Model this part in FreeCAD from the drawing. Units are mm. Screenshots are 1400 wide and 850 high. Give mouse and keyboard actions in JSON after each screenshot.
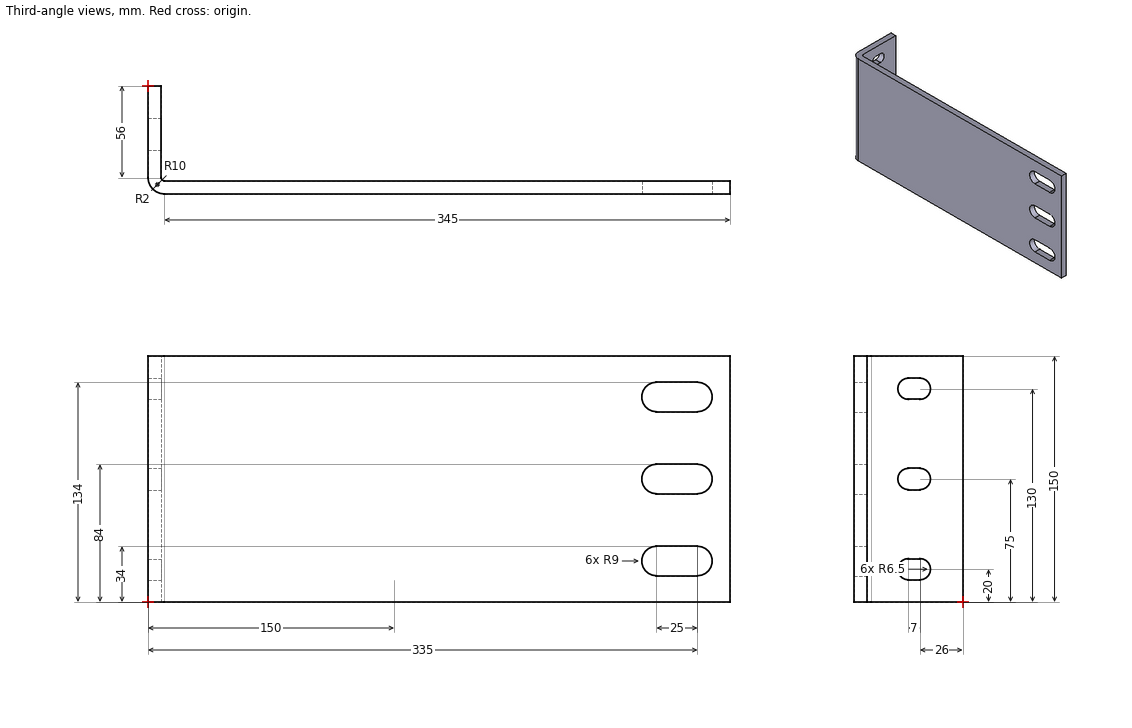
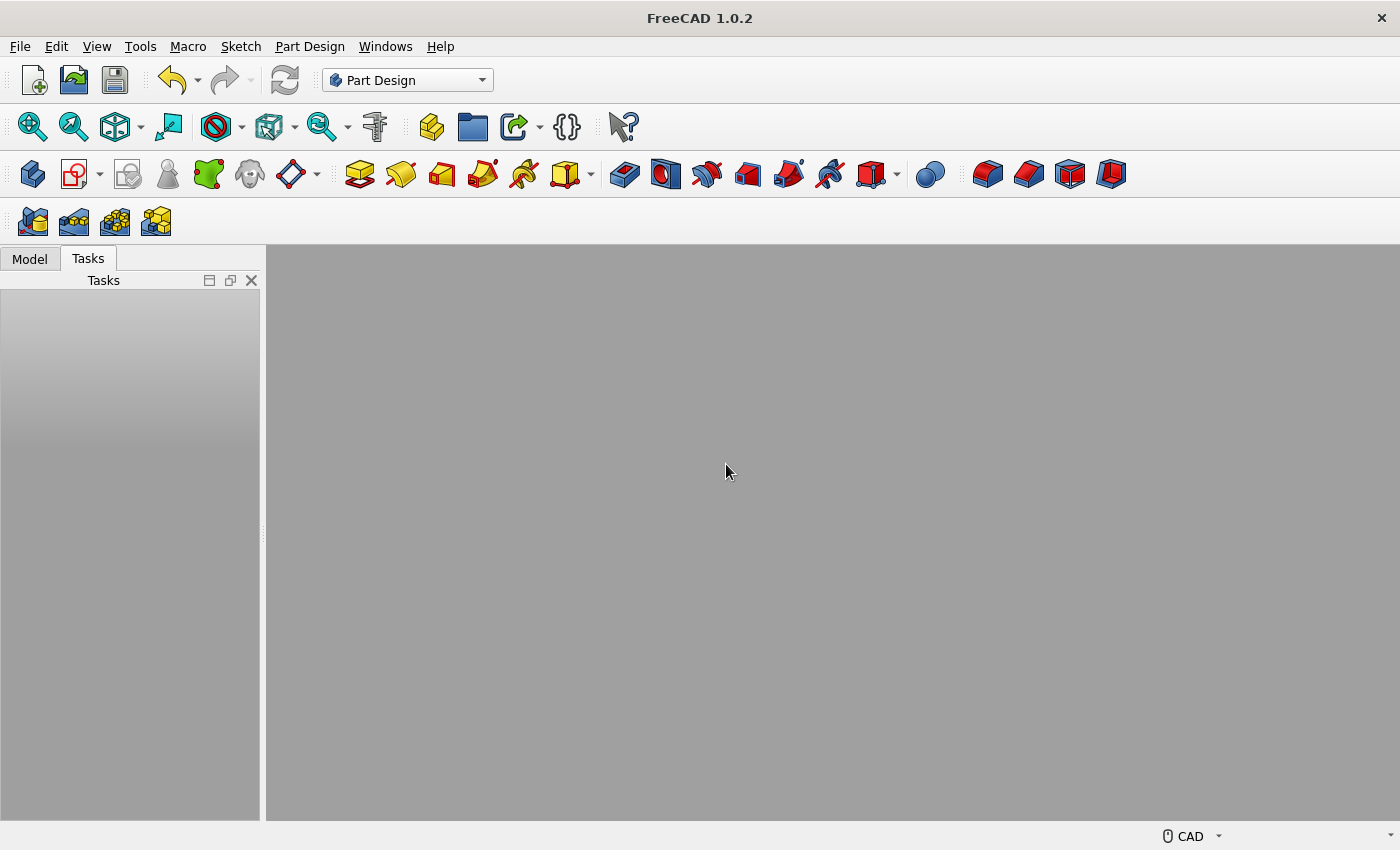
{"action": "left_click", "coordinate": [33, 80]}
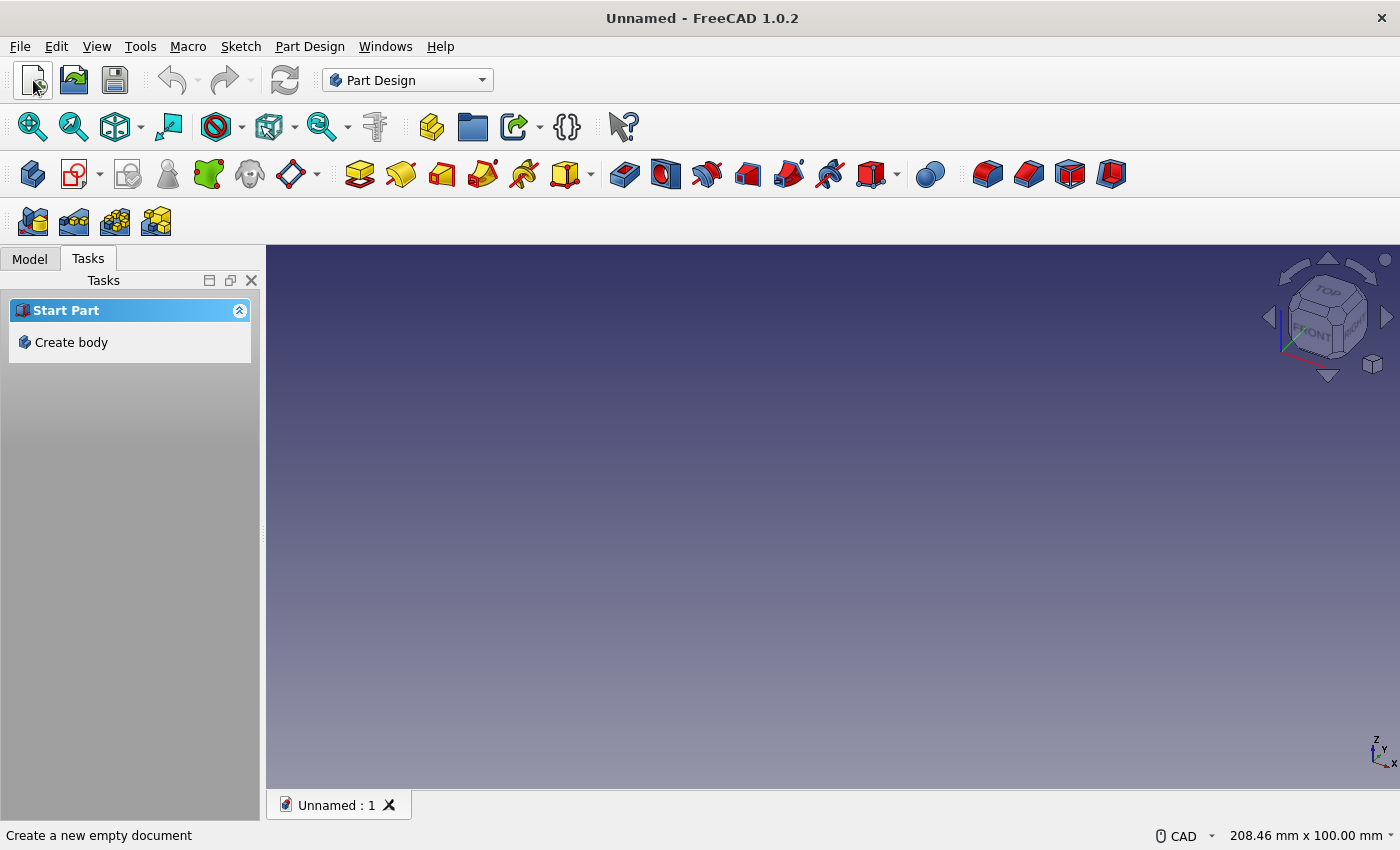
{"action": "left_click", "coordinate": [74, 174]}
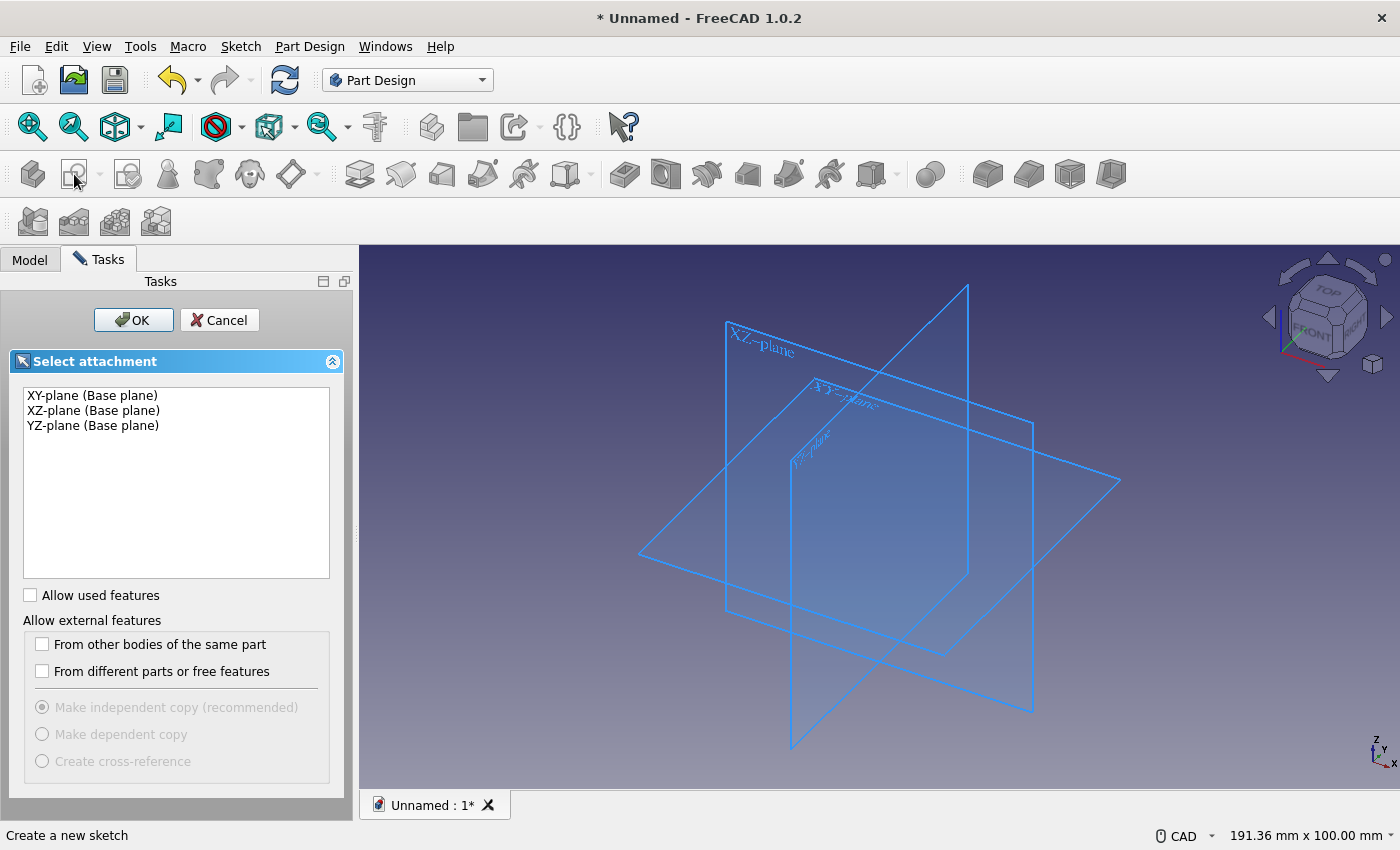
{"action": "left_click", "coordinate": [84, 396]}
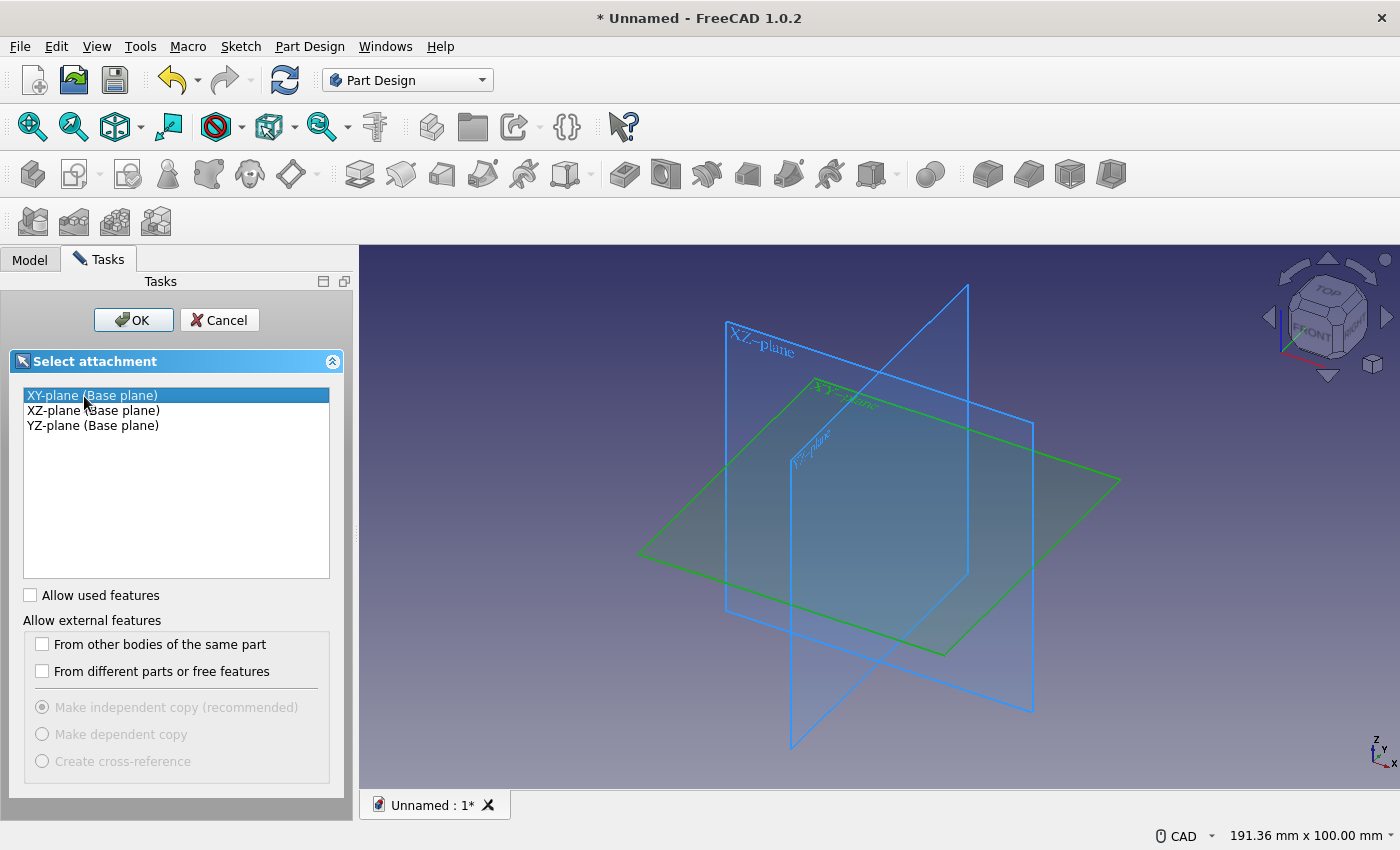
{"action": "left_click", "coordinate": [134, 320]}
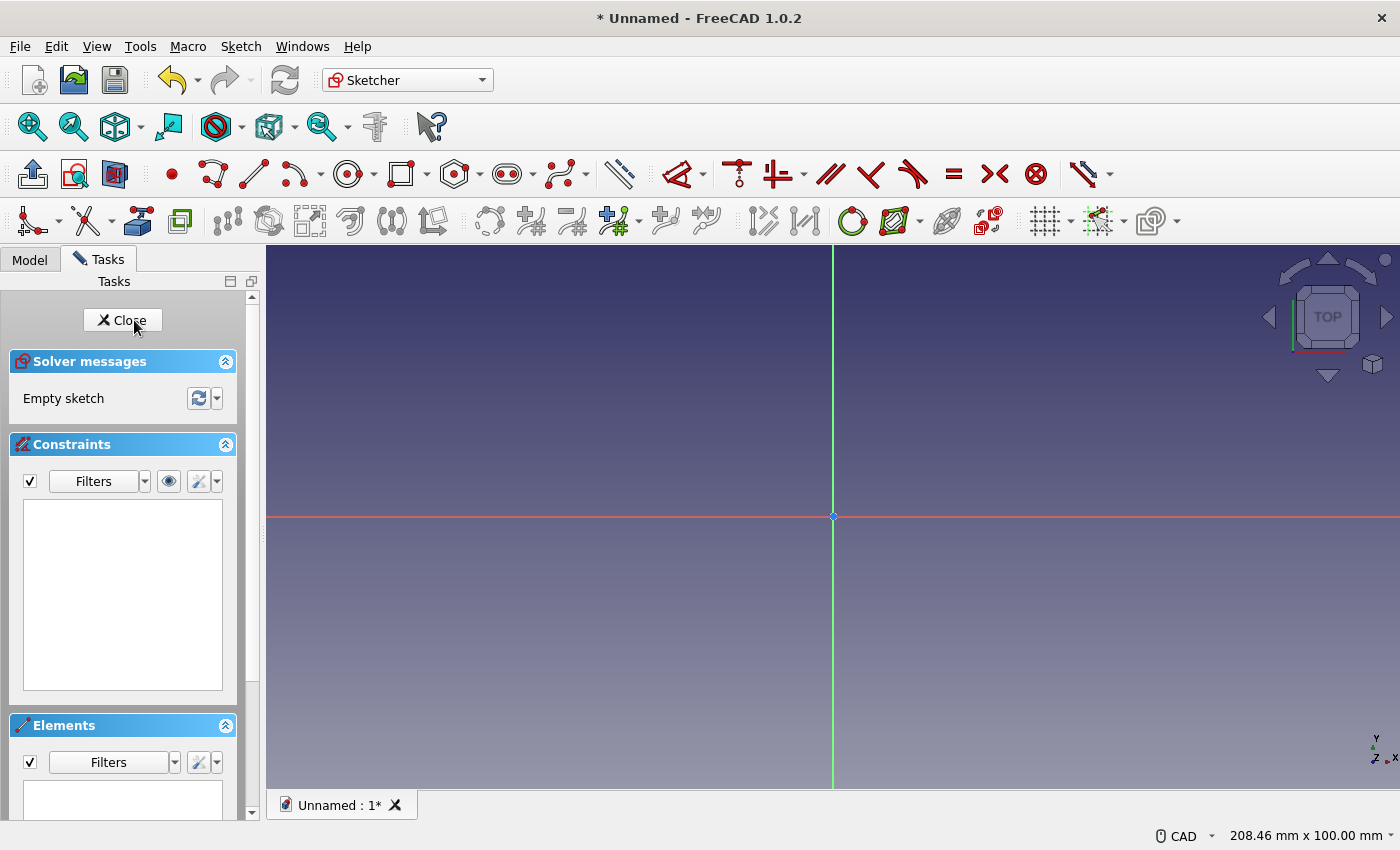
{"action": "scroll", "coordinate": [294, 413], "scroll_direction": "down", "scroll_amount": 5}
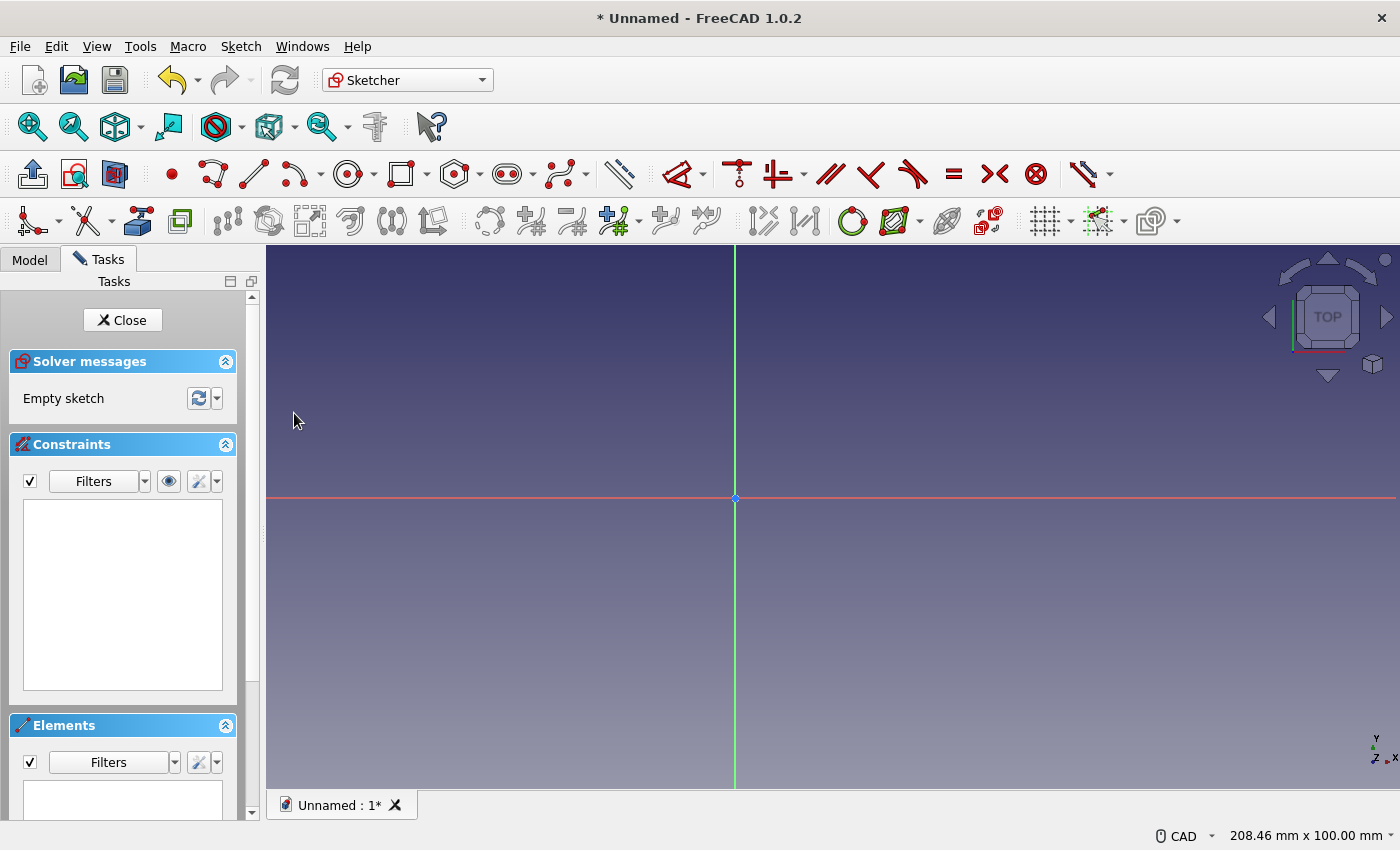
{"action": "left_click", "coordinate": [213, 174]}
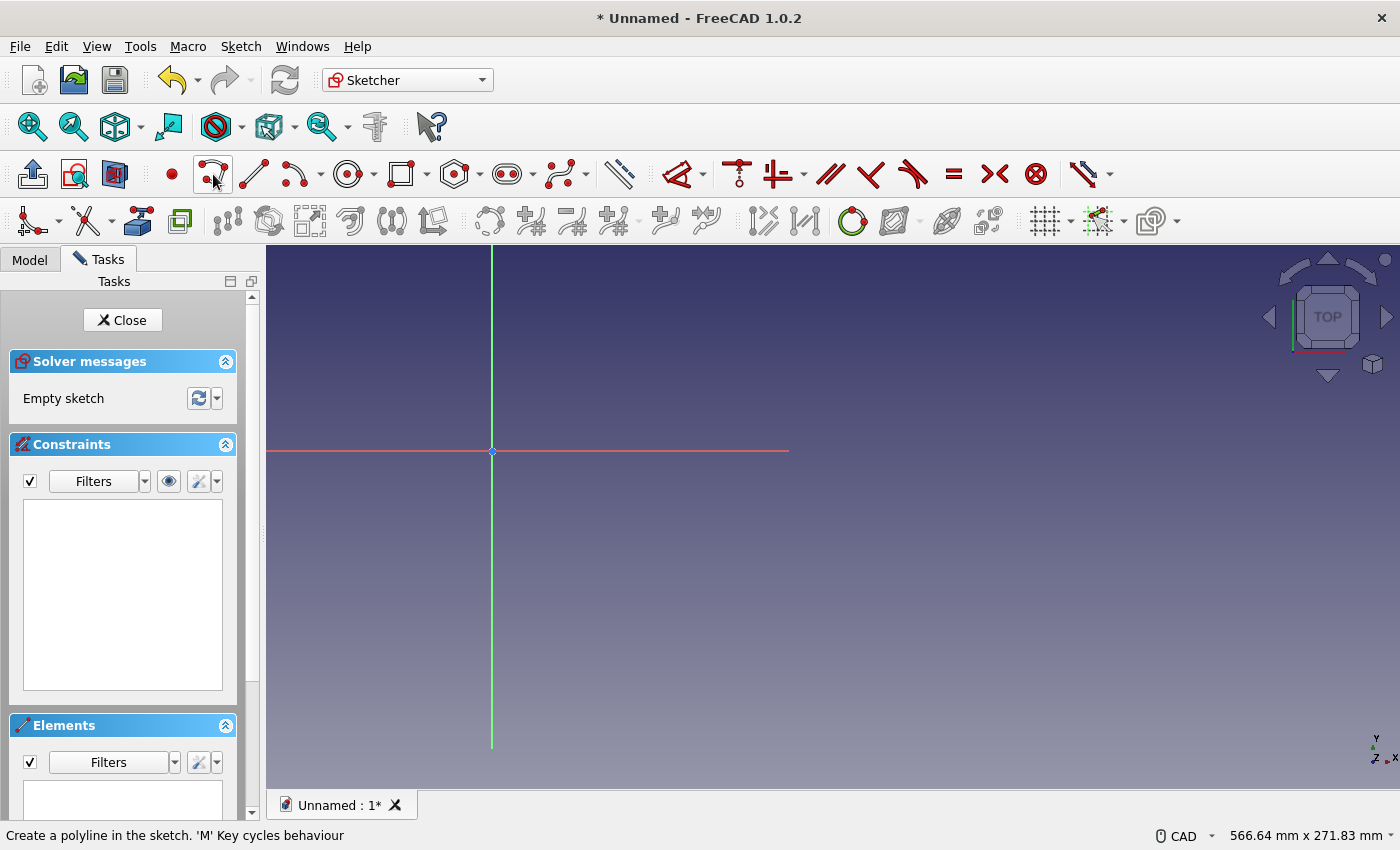
{"action": "left_click", "coordinate": [512, 584]}
{"action": "left_click", "coordinate": [1203, 584]}
{"action": "left_click", "coordinate": [1203, 568]}
{"action": "left_click", "coordinate": [512, 568]}
{"action": "right_click", "coordinate": [512, 568]}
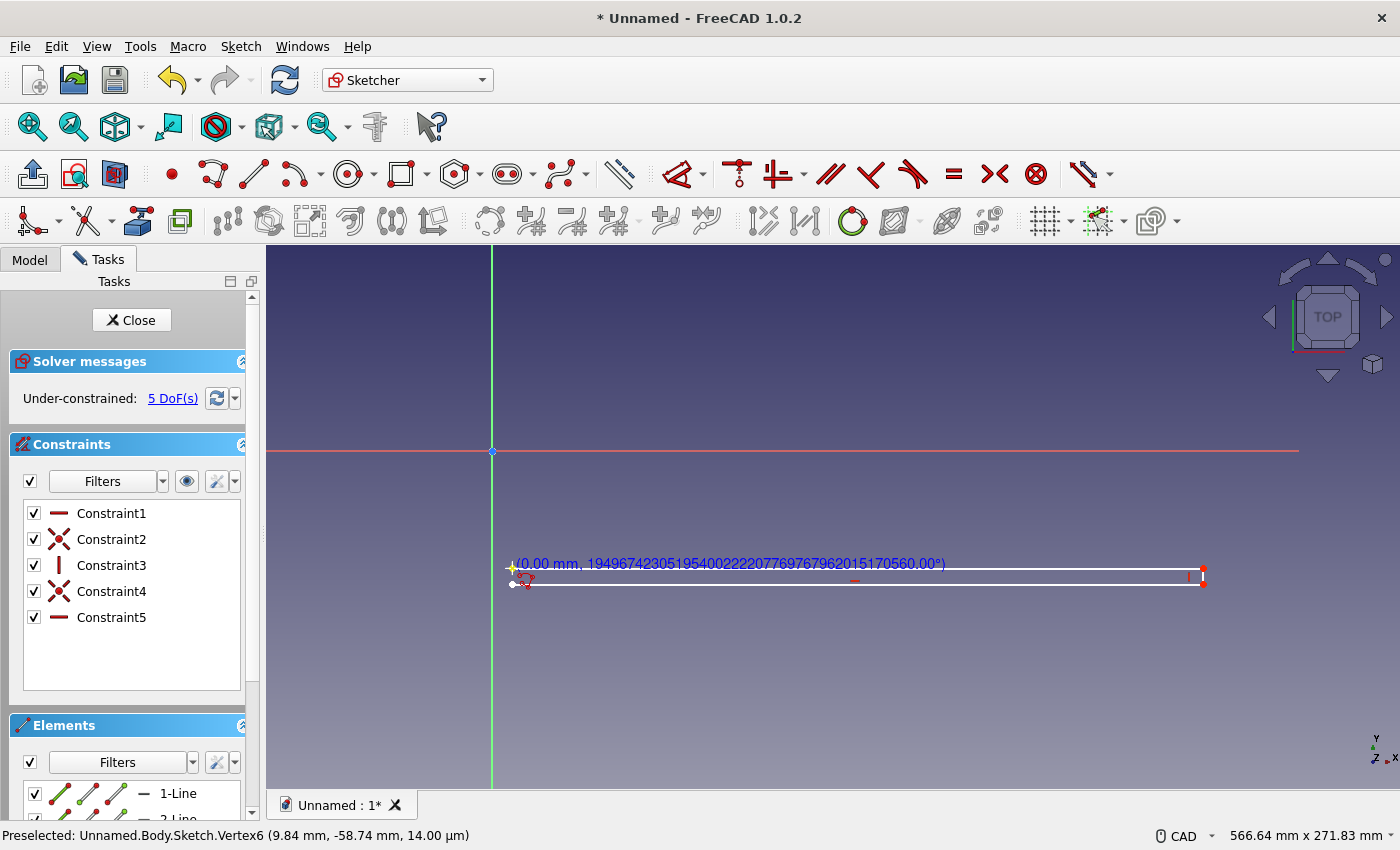
{"action": "scroll", "coordinate": [508, 564], "scroll_direction": "up", "scroll_amount": 6}